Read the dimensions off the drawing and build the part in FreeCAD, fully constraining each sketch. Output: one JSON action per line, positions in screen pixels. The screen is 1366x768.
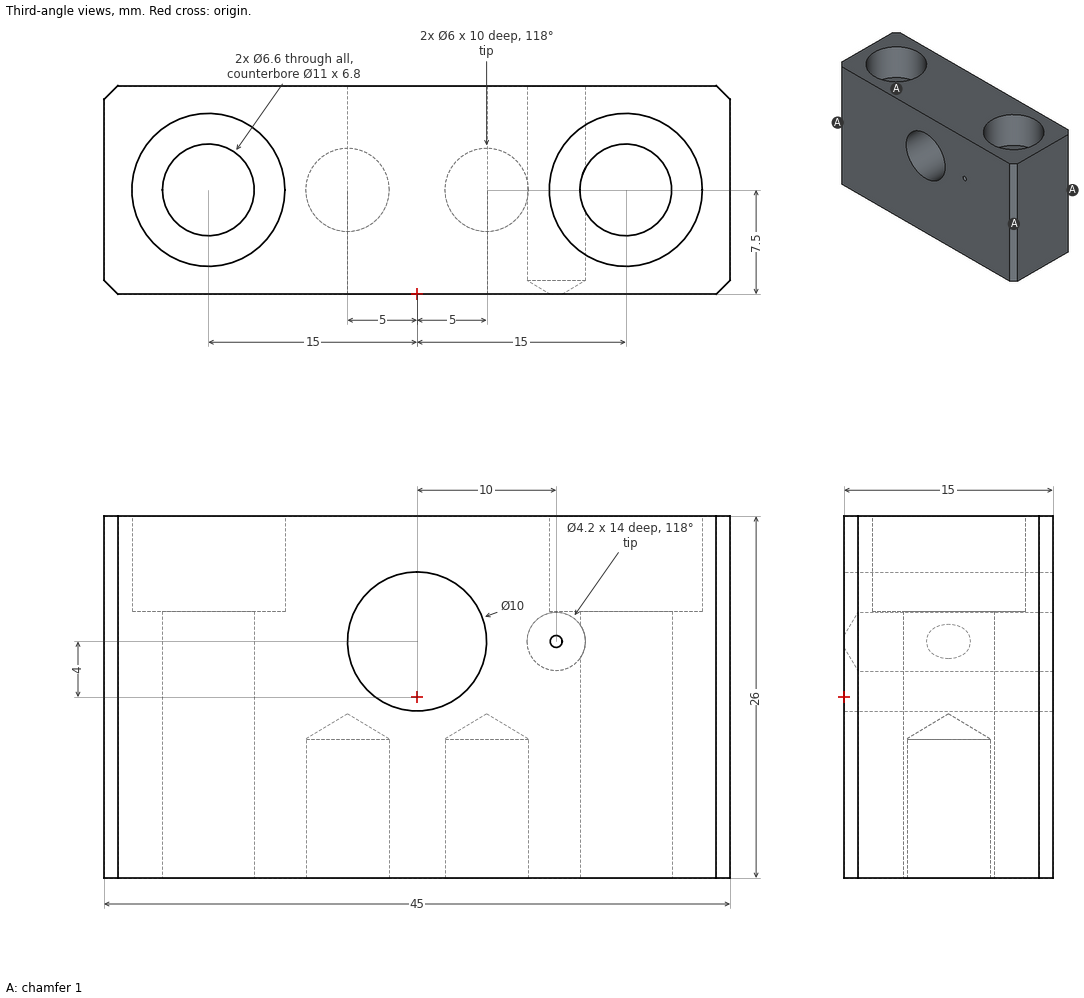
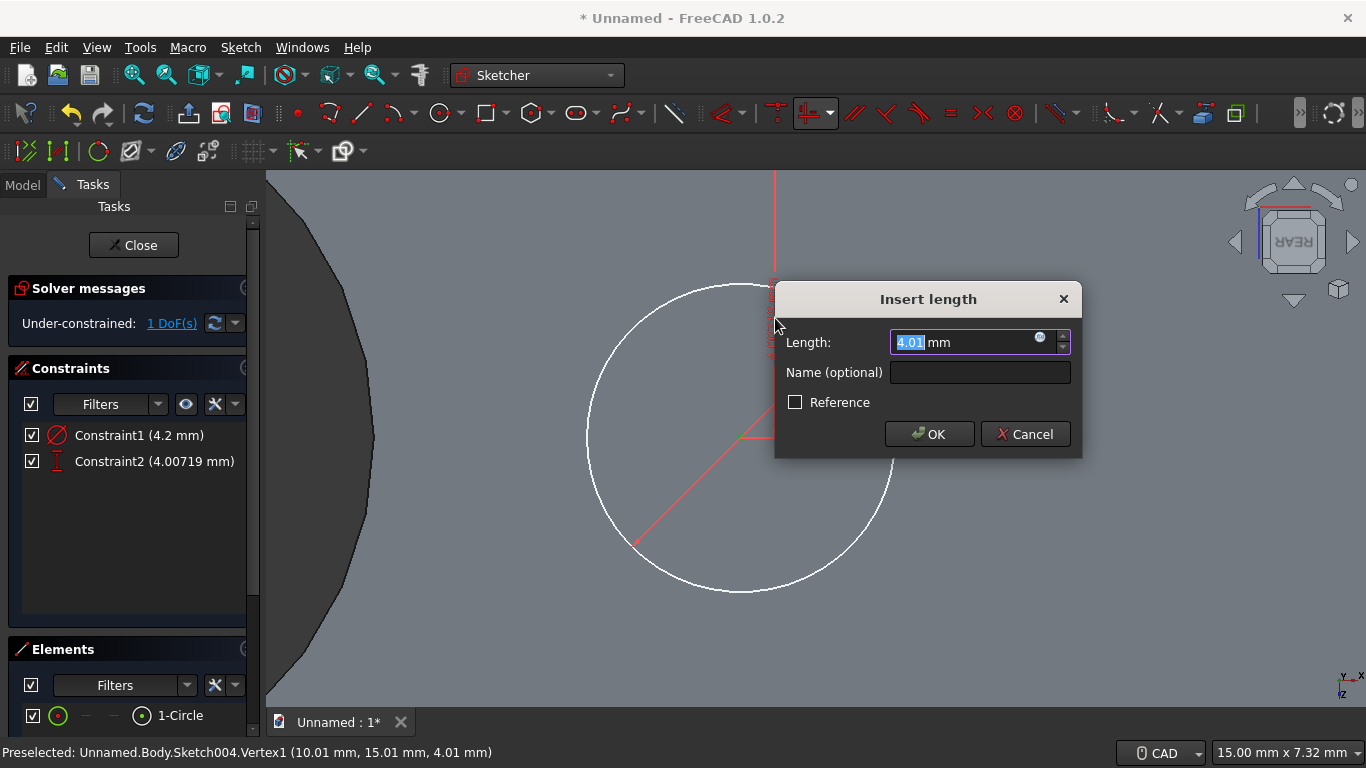
{"action": "type", "text": "4"}
{"action": "key", "text": "Return"}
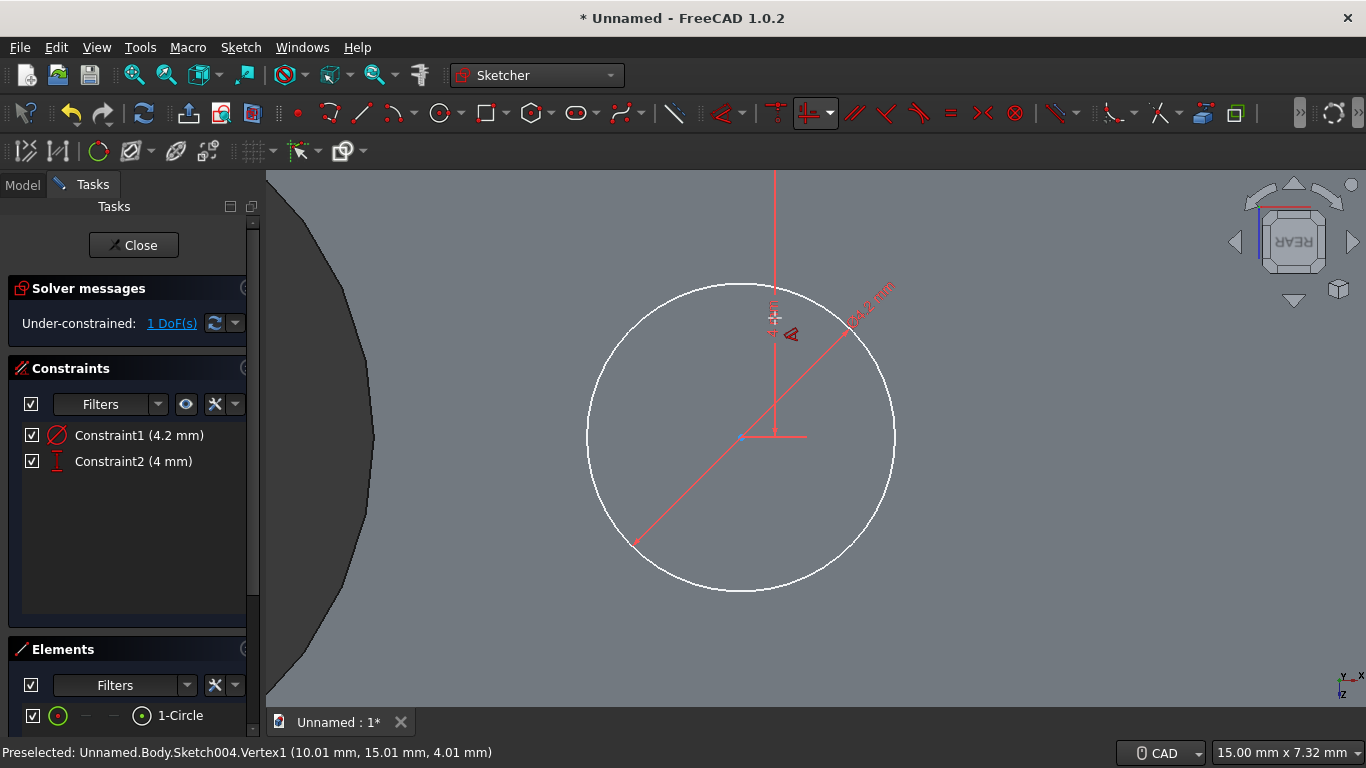
{"action": "left_click", "coordinate": [741, 437]}
{"action": "left_click", "coordinate": [518, 471]}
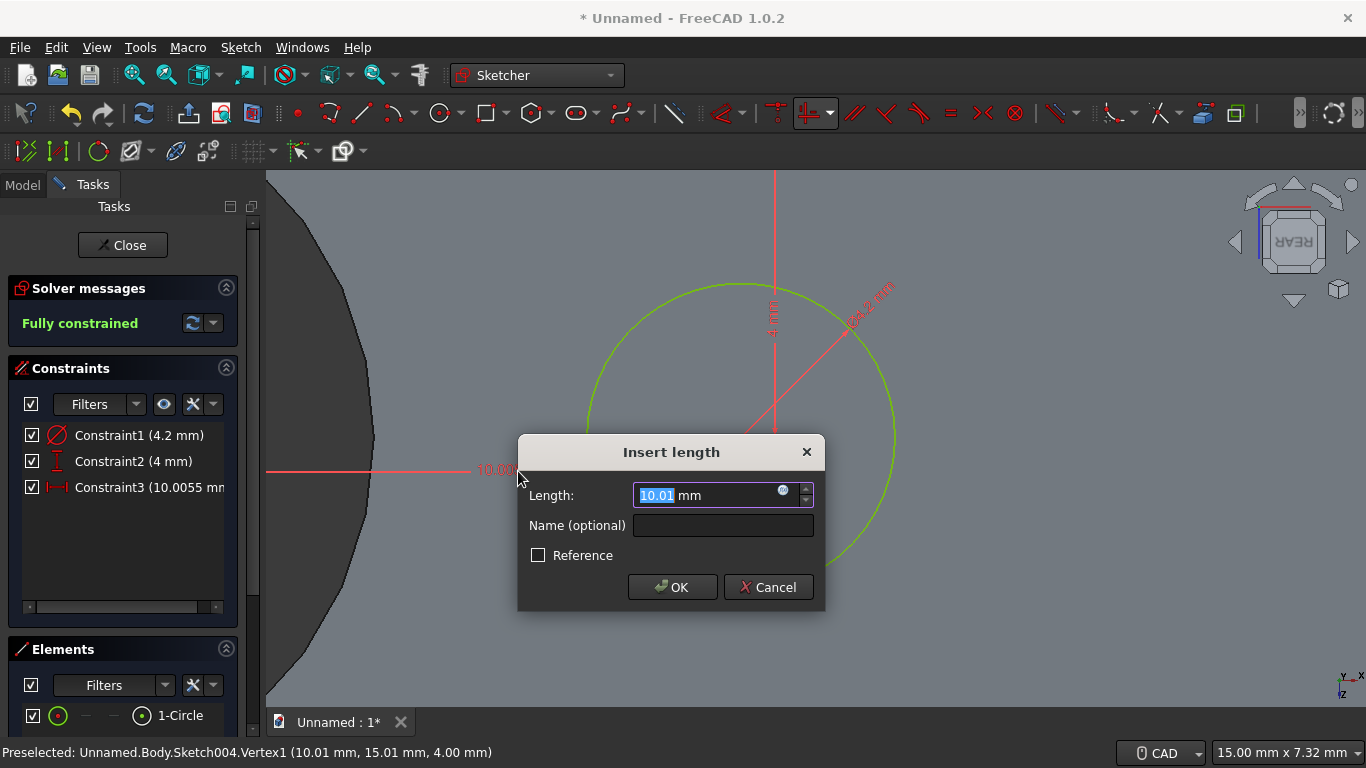
{"action": "type", "text": "10"}
{"action": "key", "text": "Return"}
{"action": "key", "text": "Escape"}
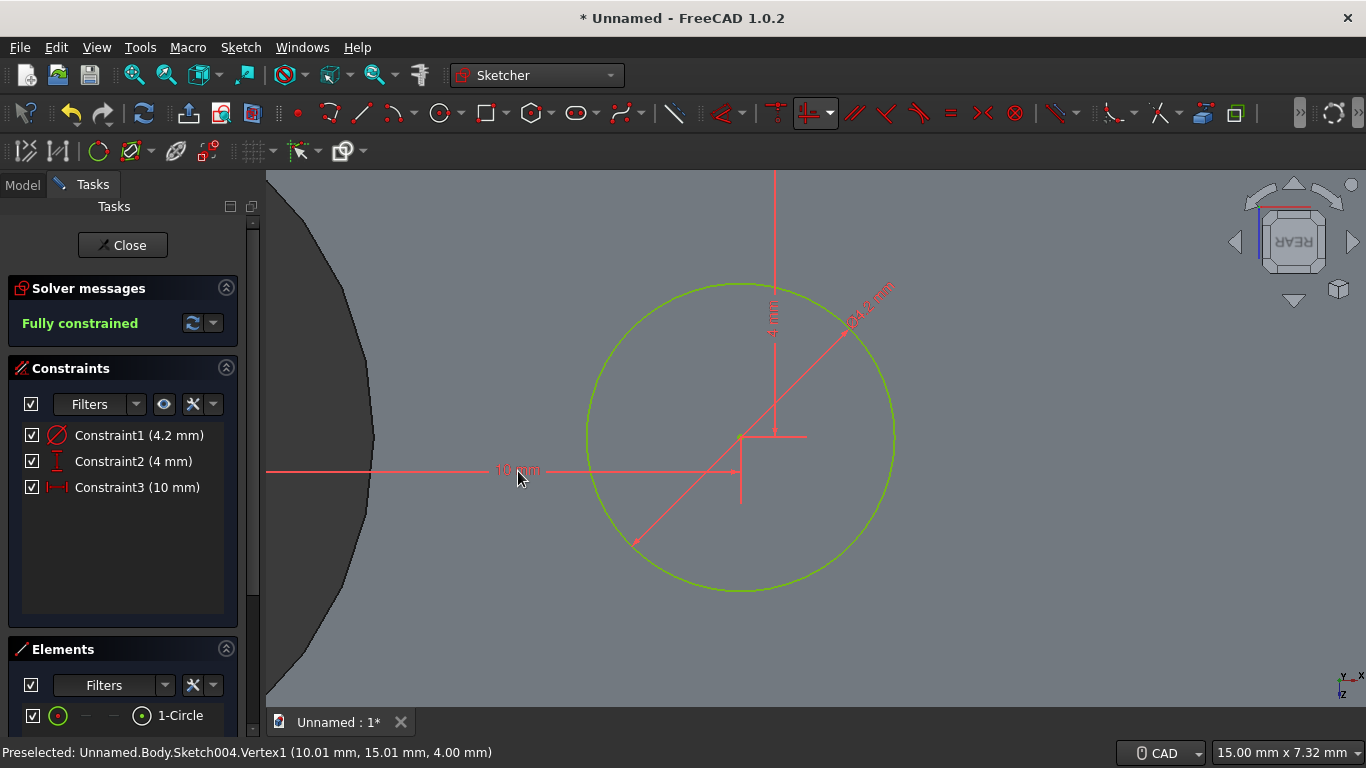
{"action": "left_click", "coordinate": [123, 245]}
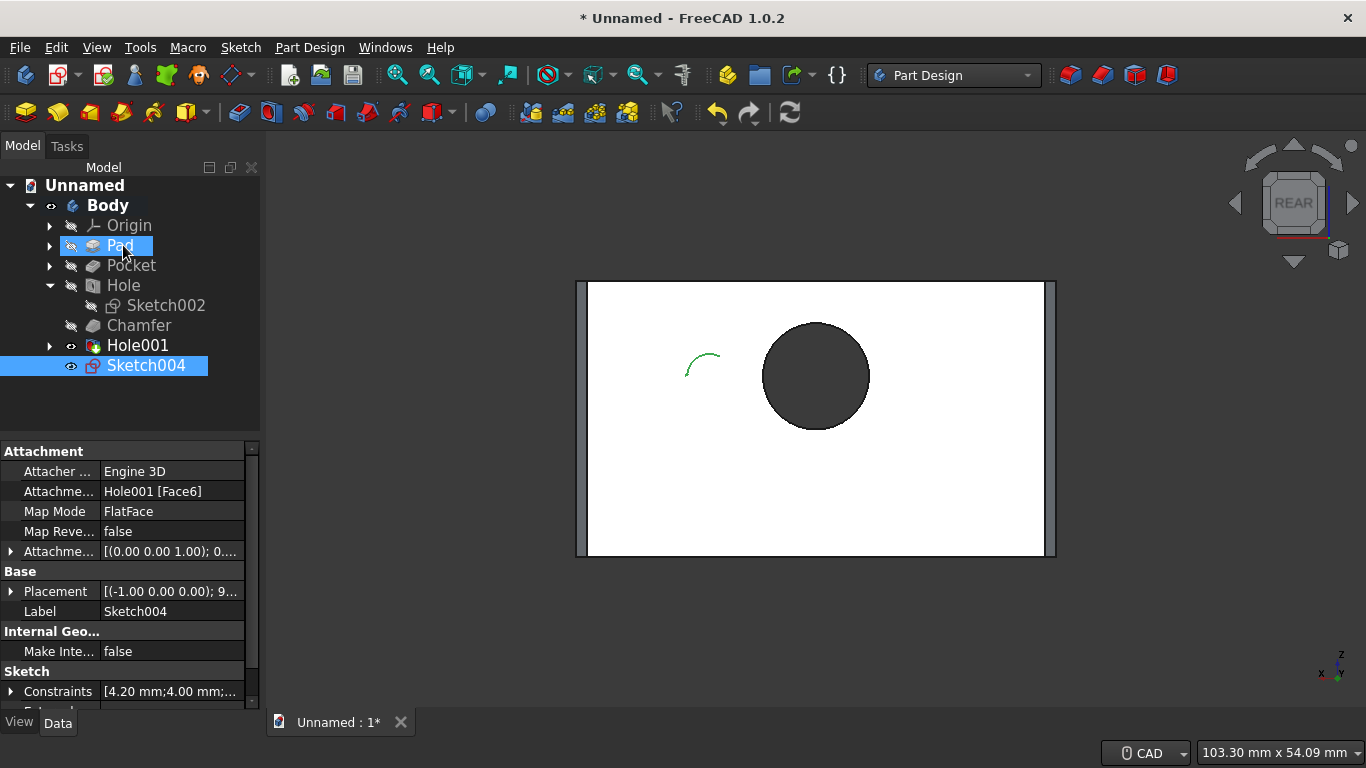
{"action": "left_click", "coordinate": [272, 112]}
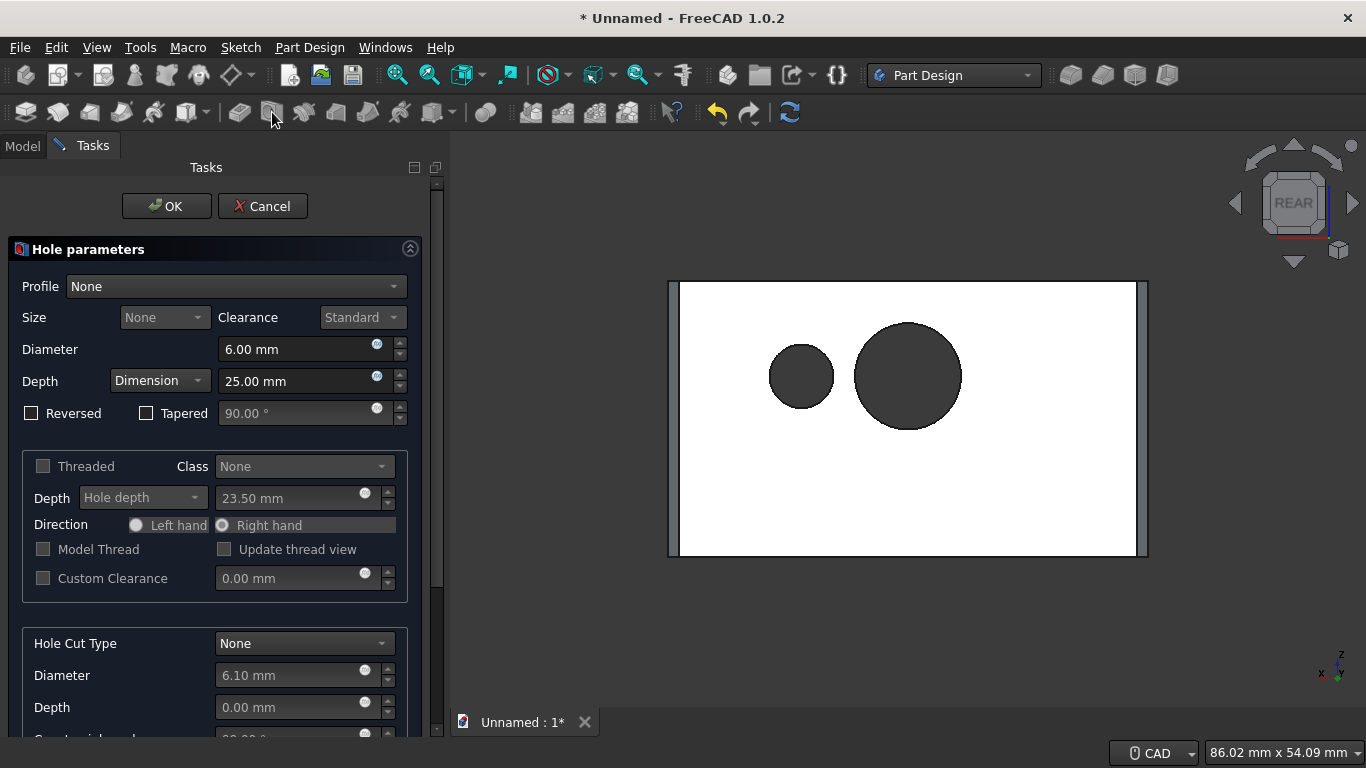
{"action": "triple_click", "coordinate": [305, 349]}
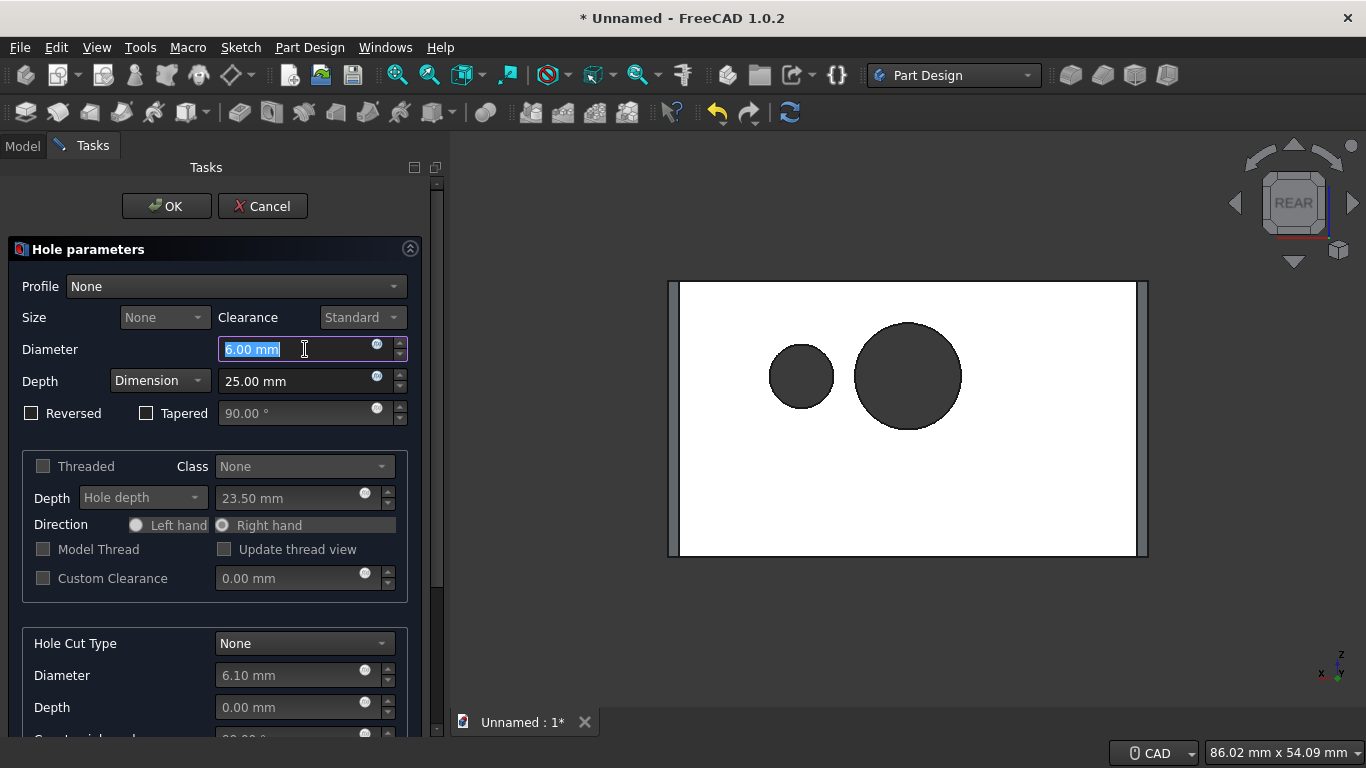
{"action": "type", "text": "4.2"}
{"action": "key", "text": "Tab"}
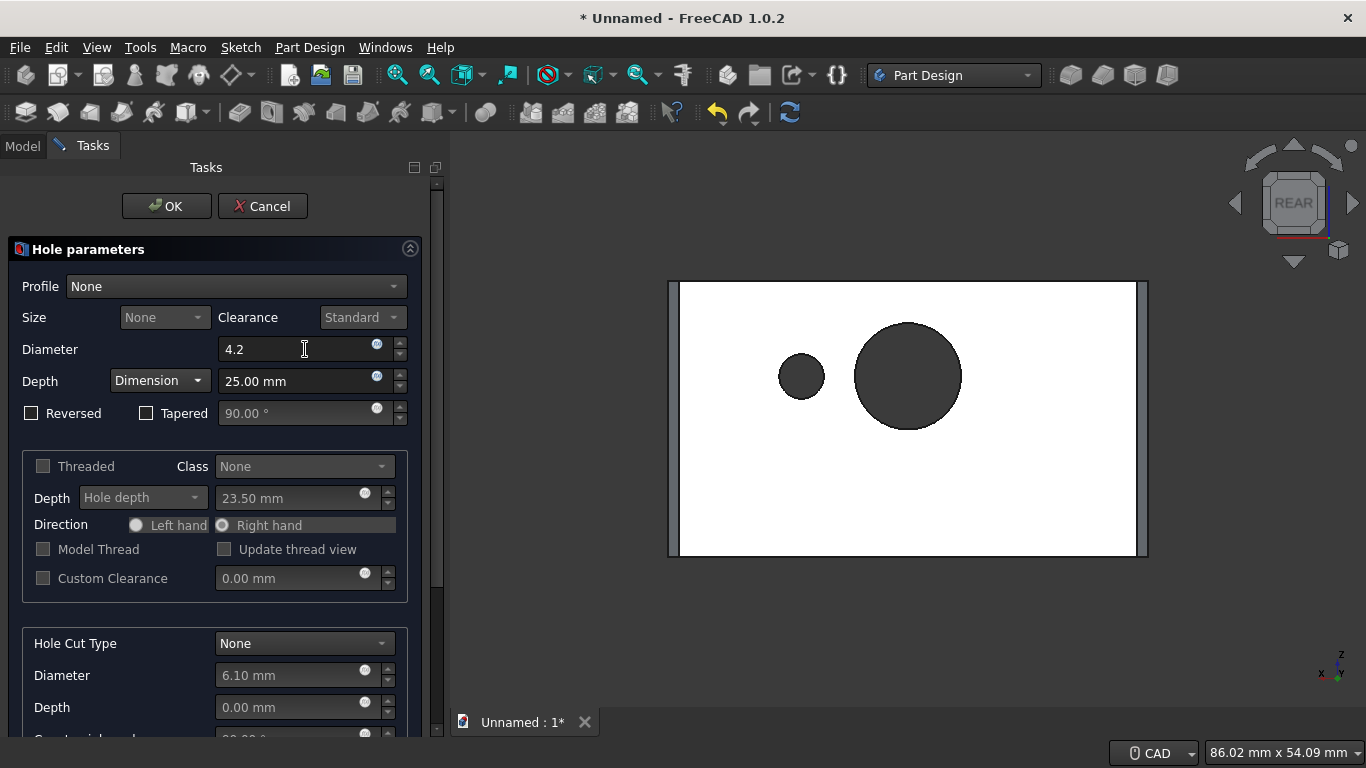
{"action": "triple_click", "coordinate": [305, 381]}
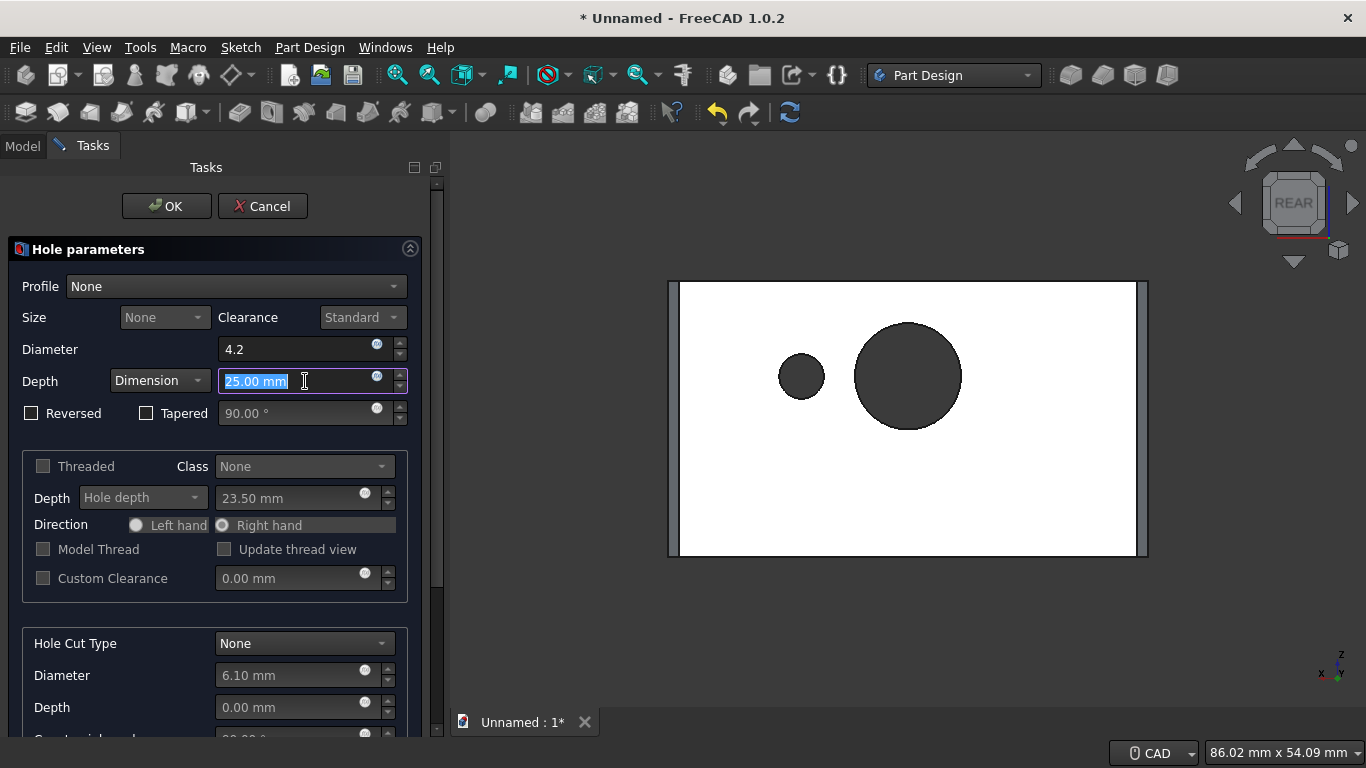
{"action": "type", "text": "14"}
{"action": "key", "text": "Tab"}